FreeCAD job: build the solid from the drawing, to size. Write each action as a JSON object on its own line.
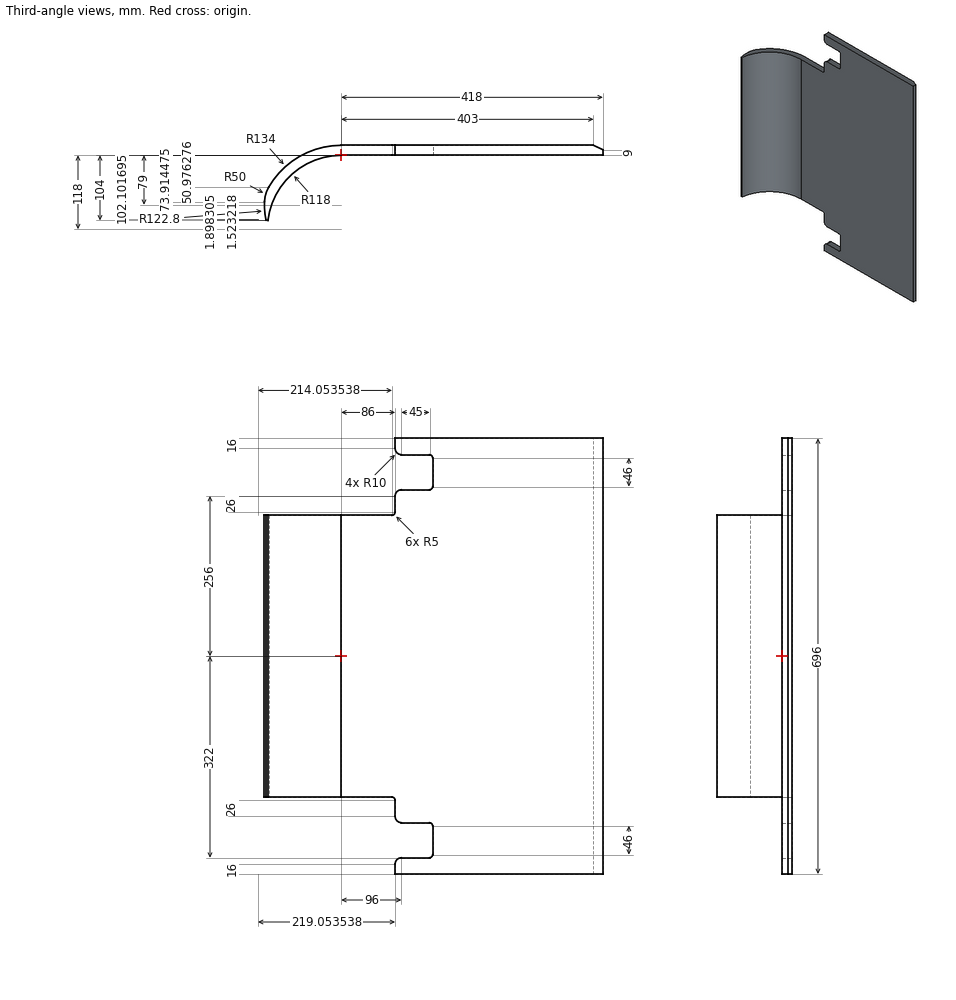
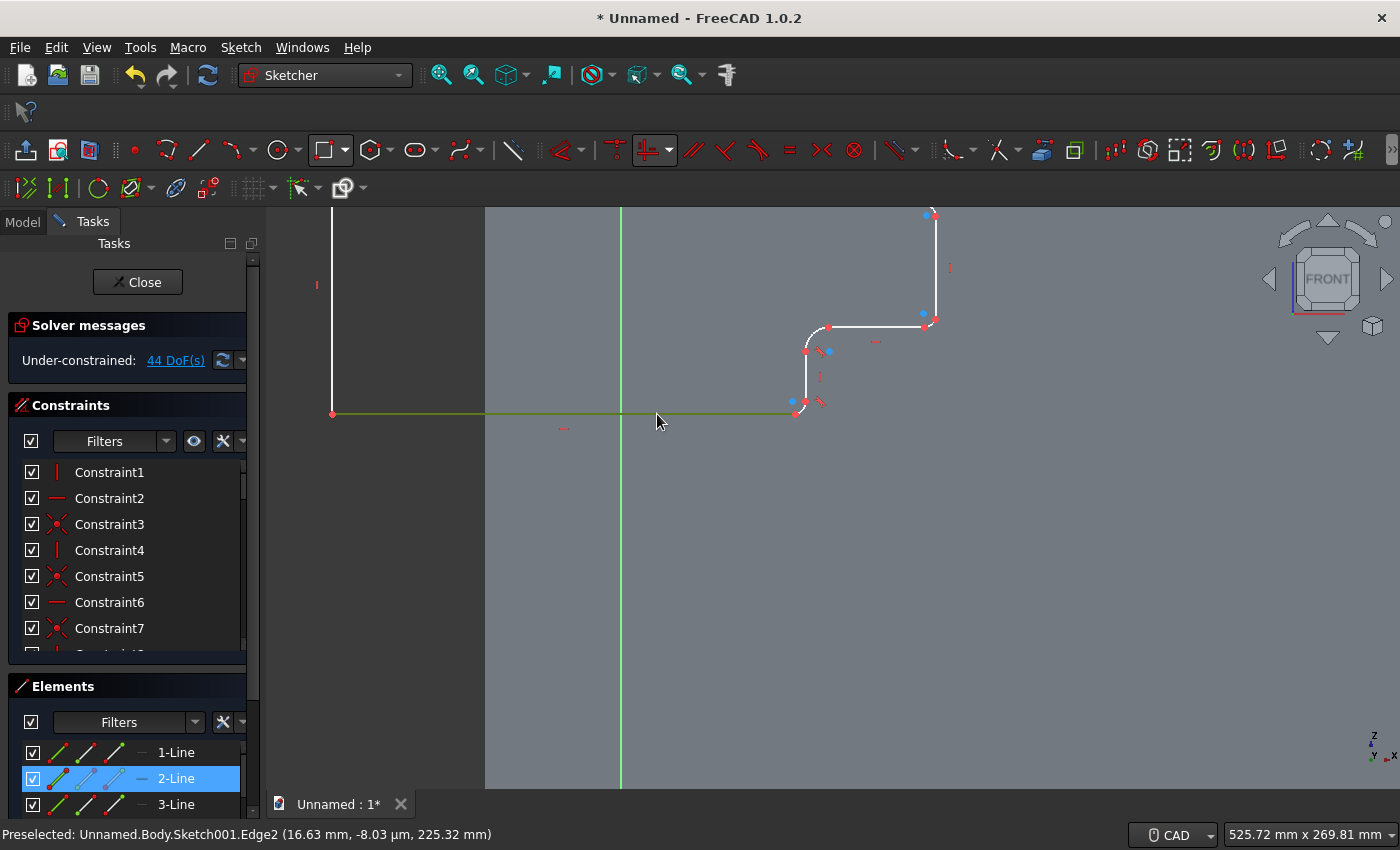
{"action": "scroll", "coordinate": [803, 409], "scroll_direction": "up", "scroll_amount": 3}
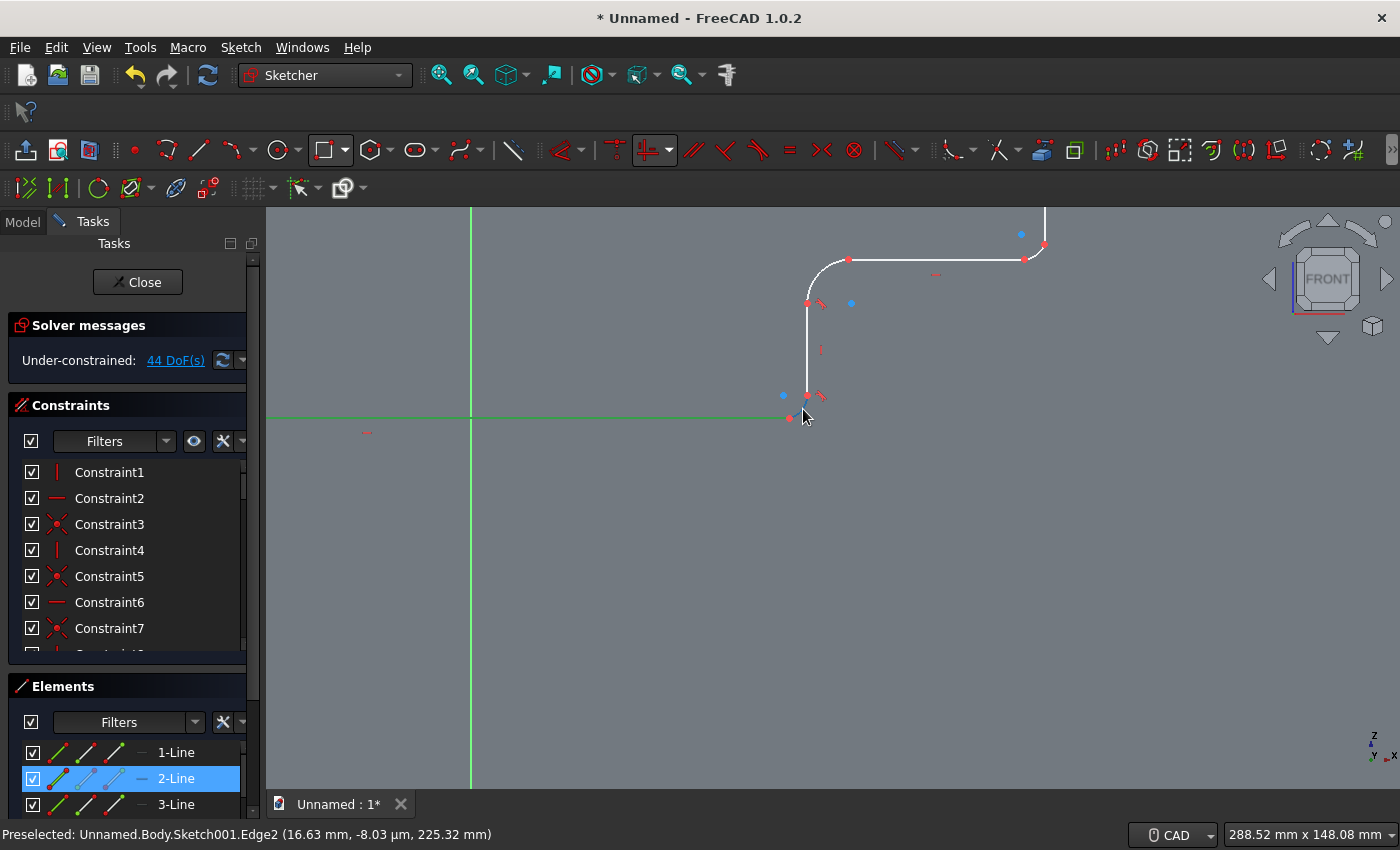
{"action": "left_click", "coordinate": [802, 410]}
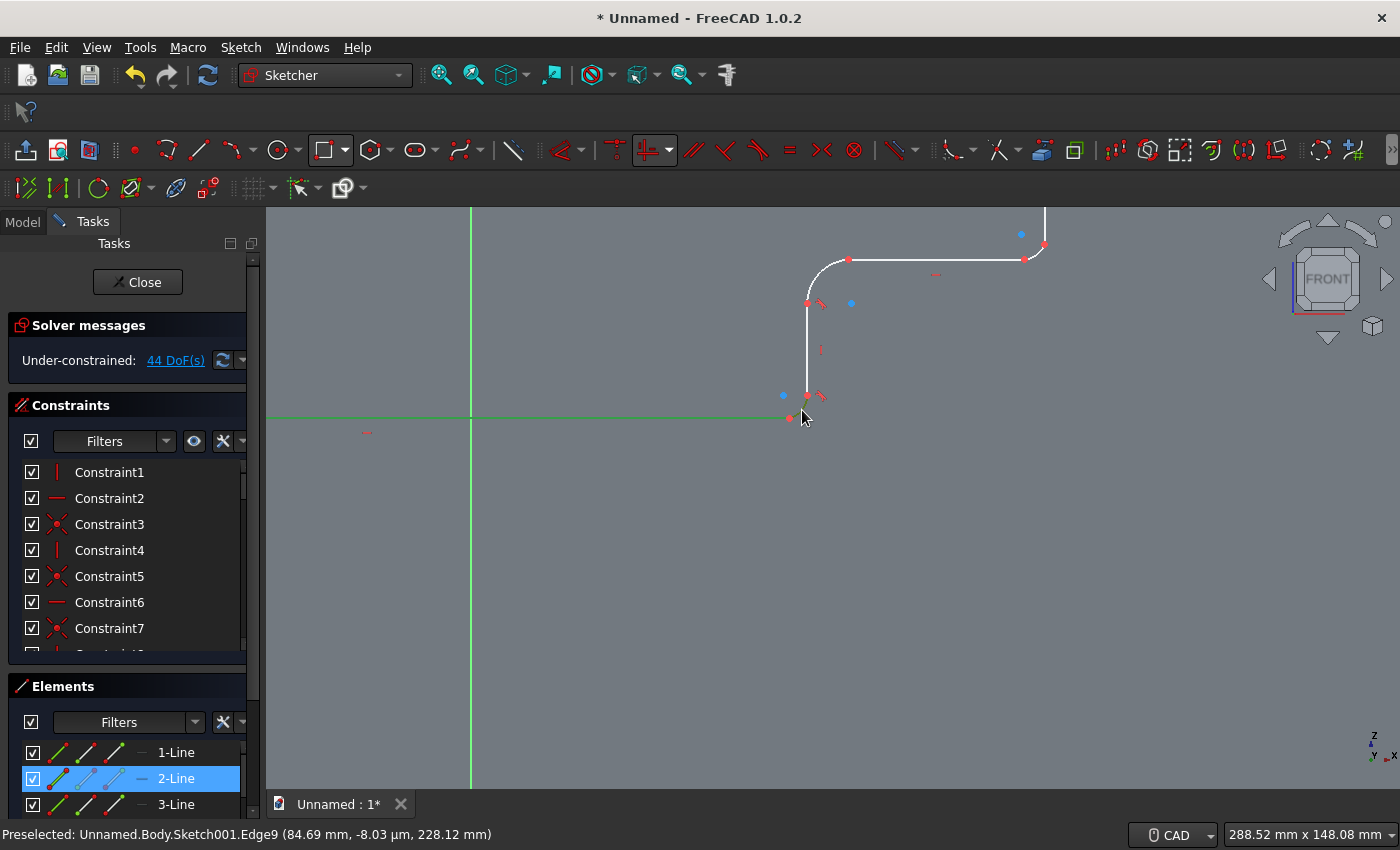
{"action": "left_click", "coordinate": [758, 150]}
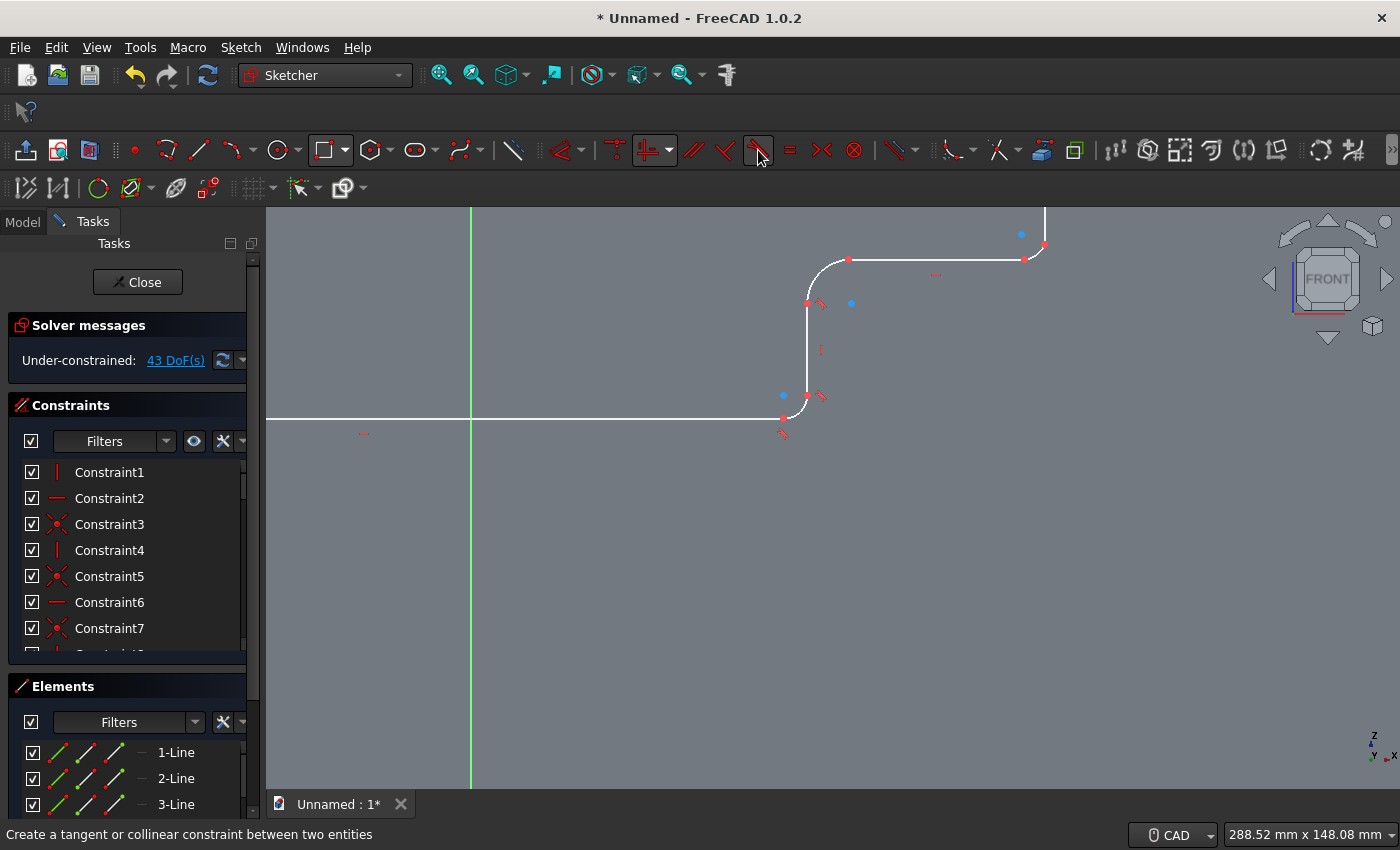
{"action": "scroll", "coordinate": [806, 372], "scroll_direction": "down", "scroll_amount": 10}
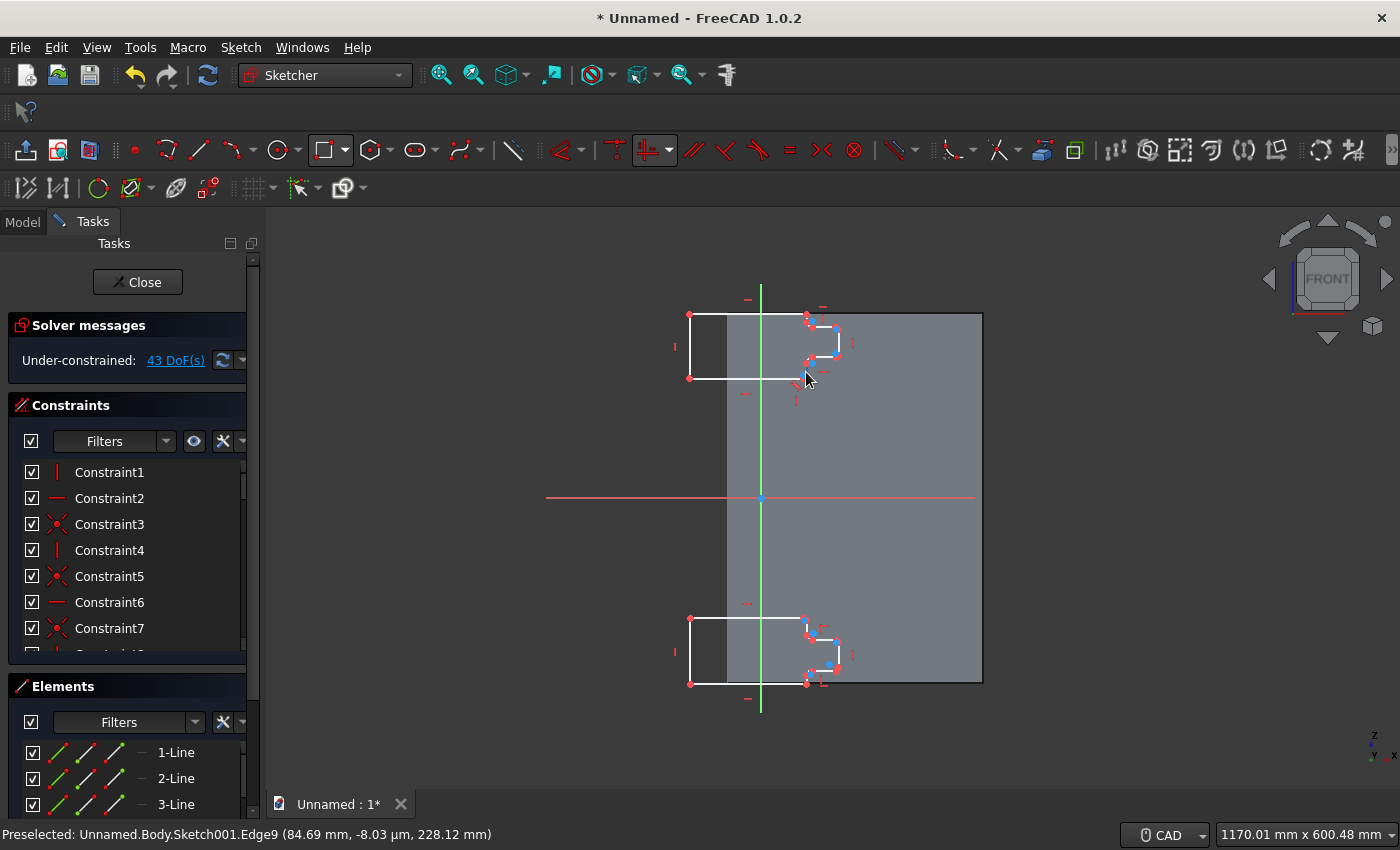
{"action": "scroll", "coordinate": [807, 317], "scroll_direction": "up", "scroll_amount": 9}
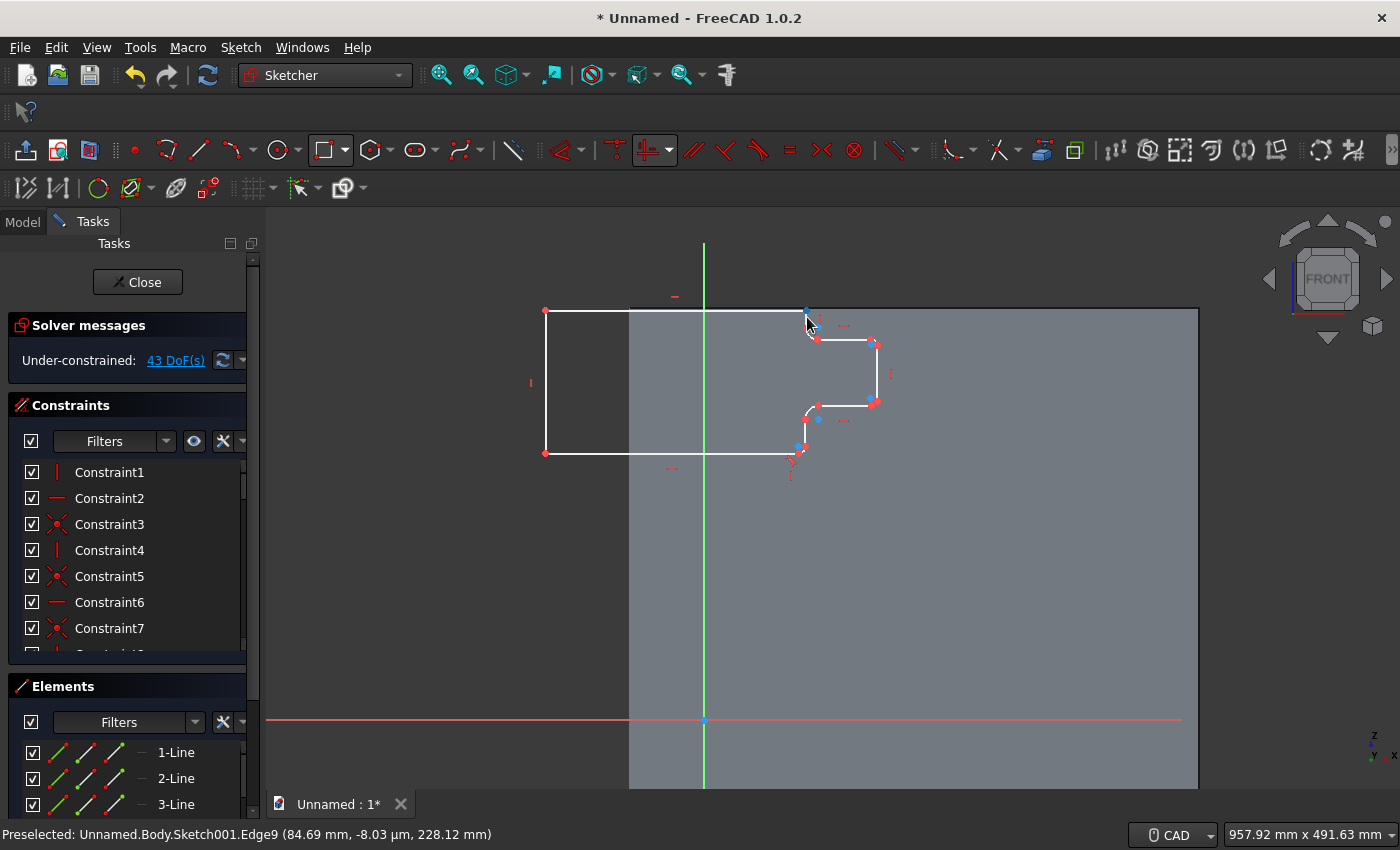
{"action": "left_click", "coordinate": [804, 315]}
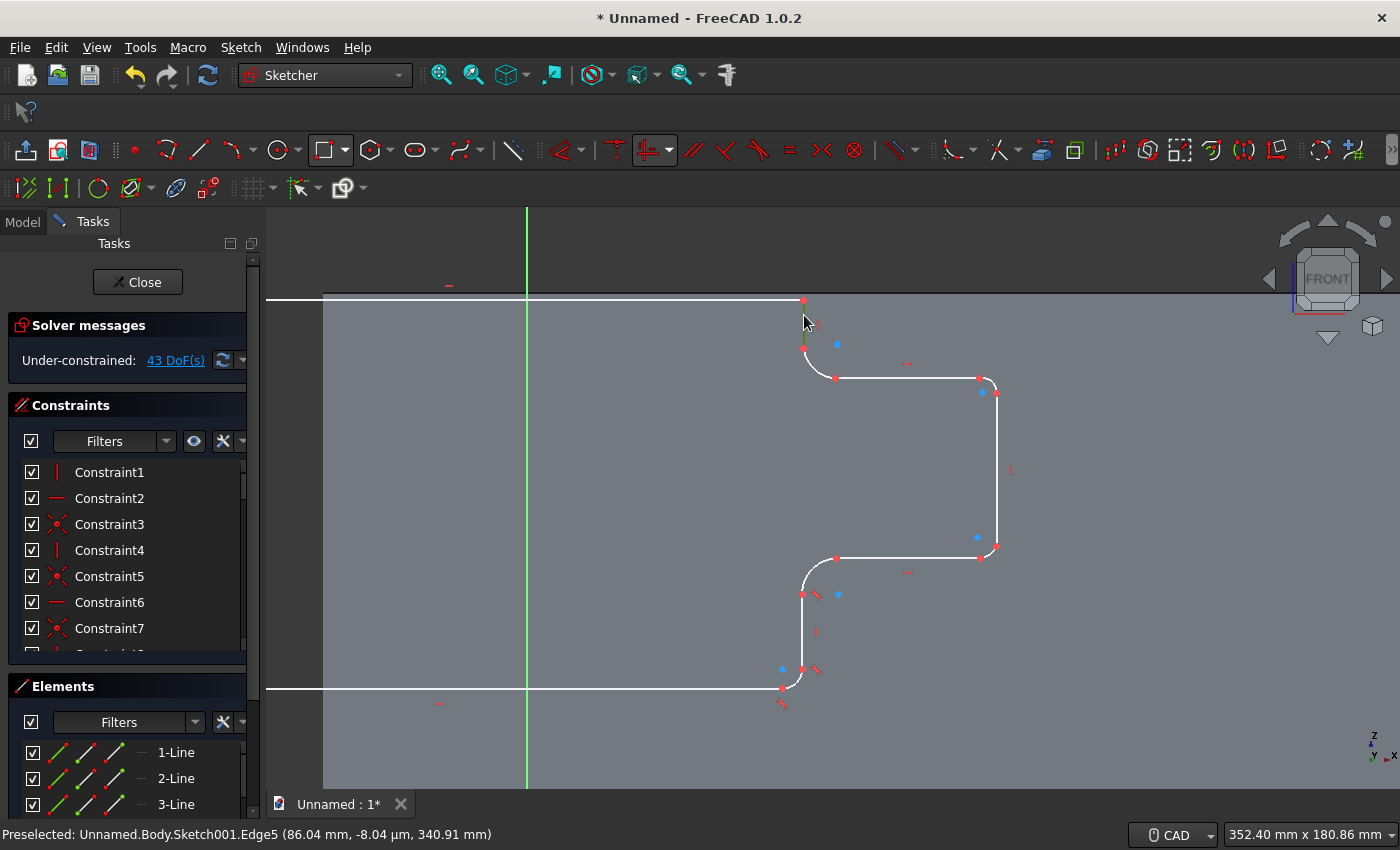
{"action": "left_click", "coordinate": [808, 362]}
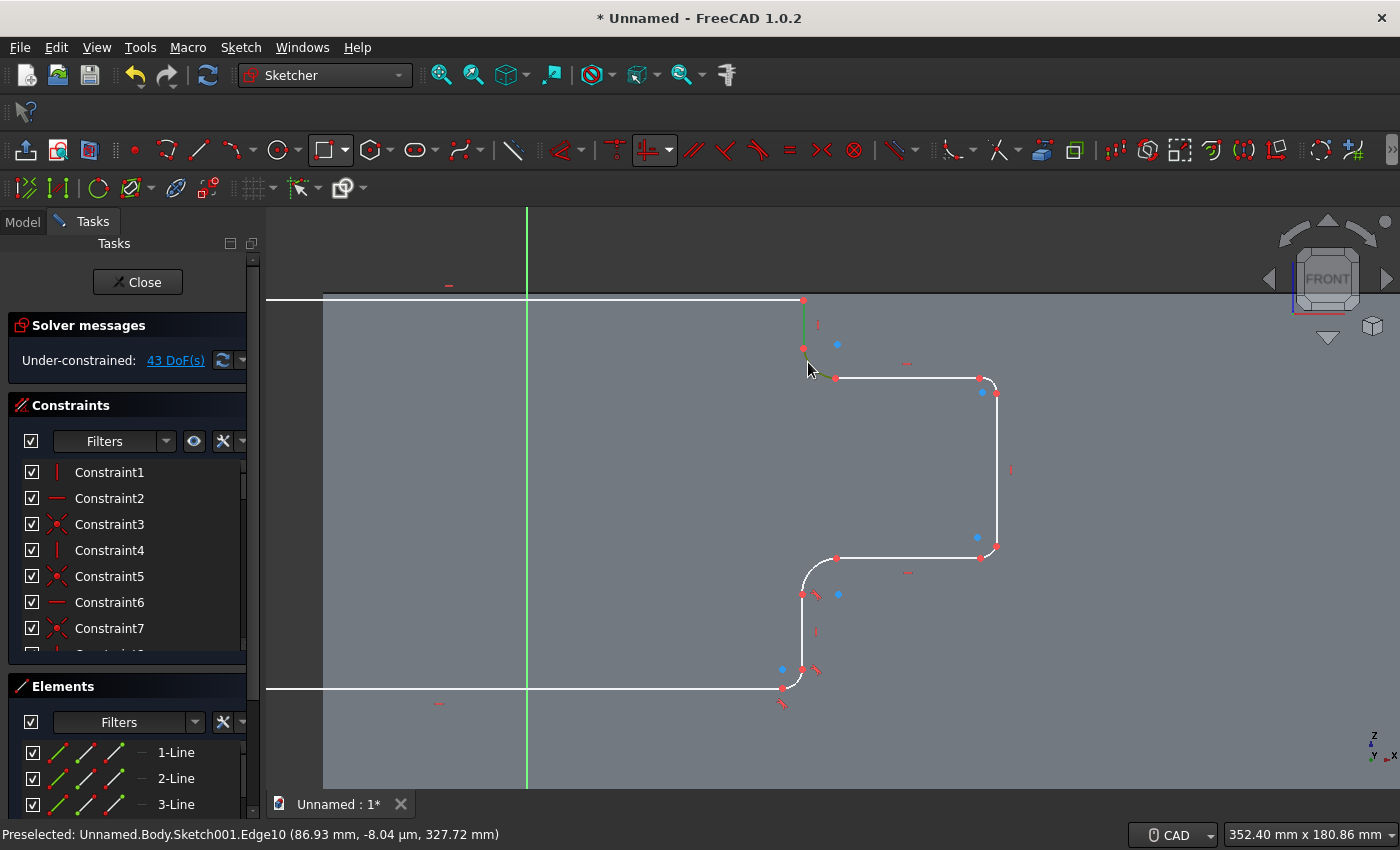
{"action": "left_click", "coordinate": [758, 150]}